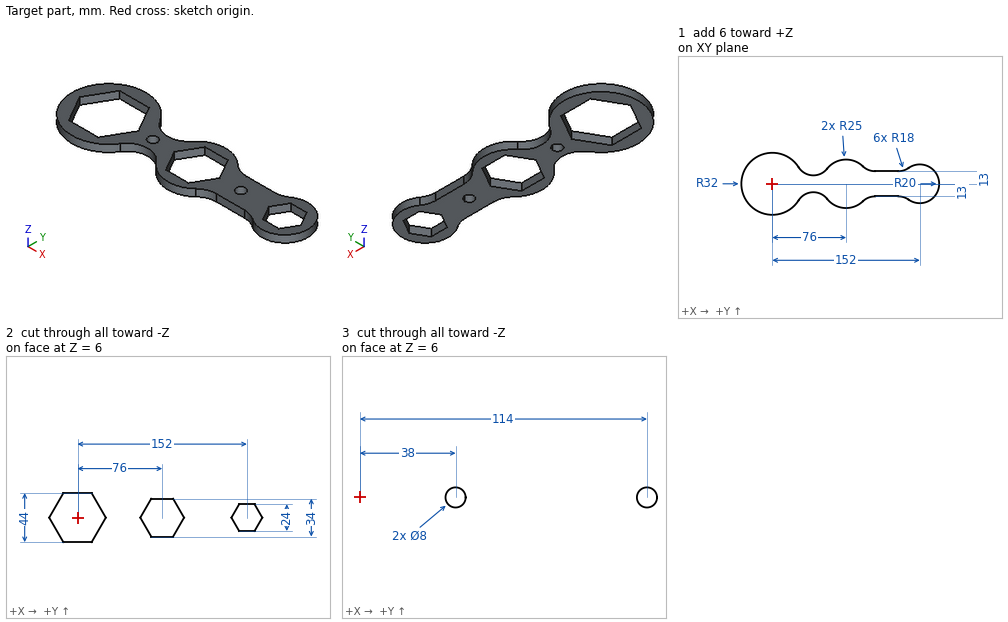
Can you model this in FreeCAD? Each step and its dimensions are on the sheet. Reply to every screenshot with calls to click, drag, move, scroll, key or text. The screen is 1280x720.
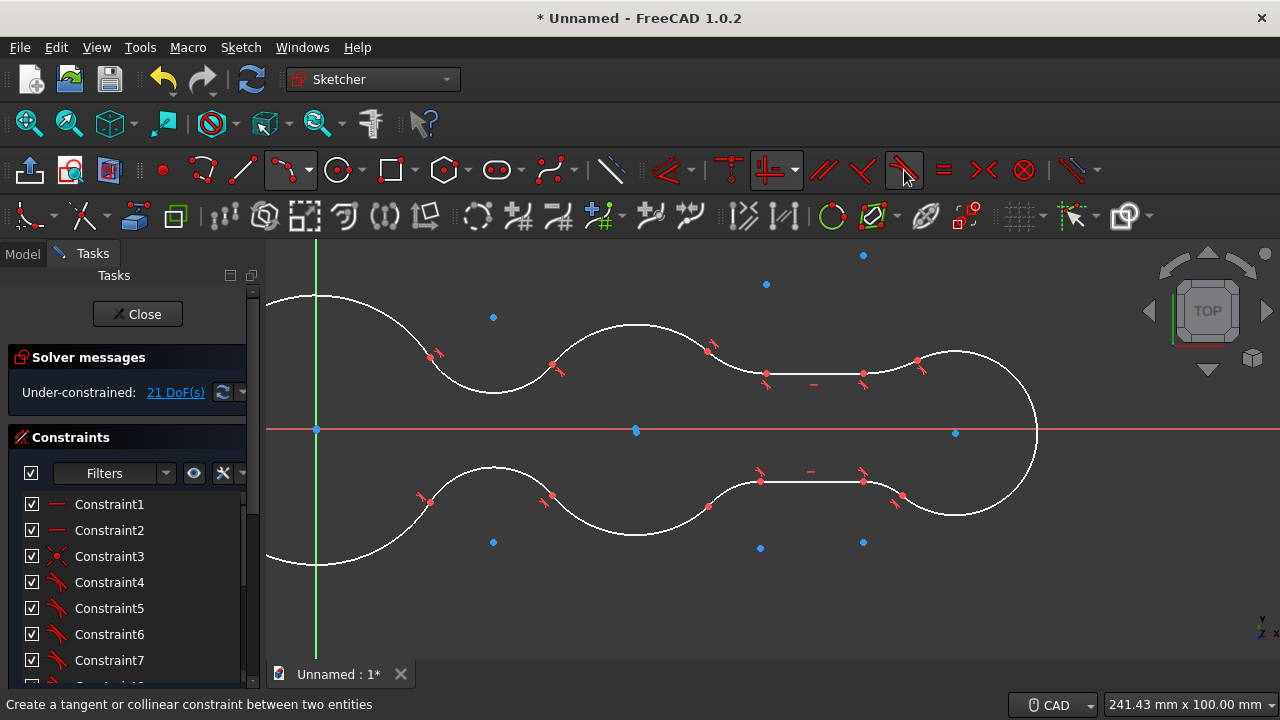
click(594, 527)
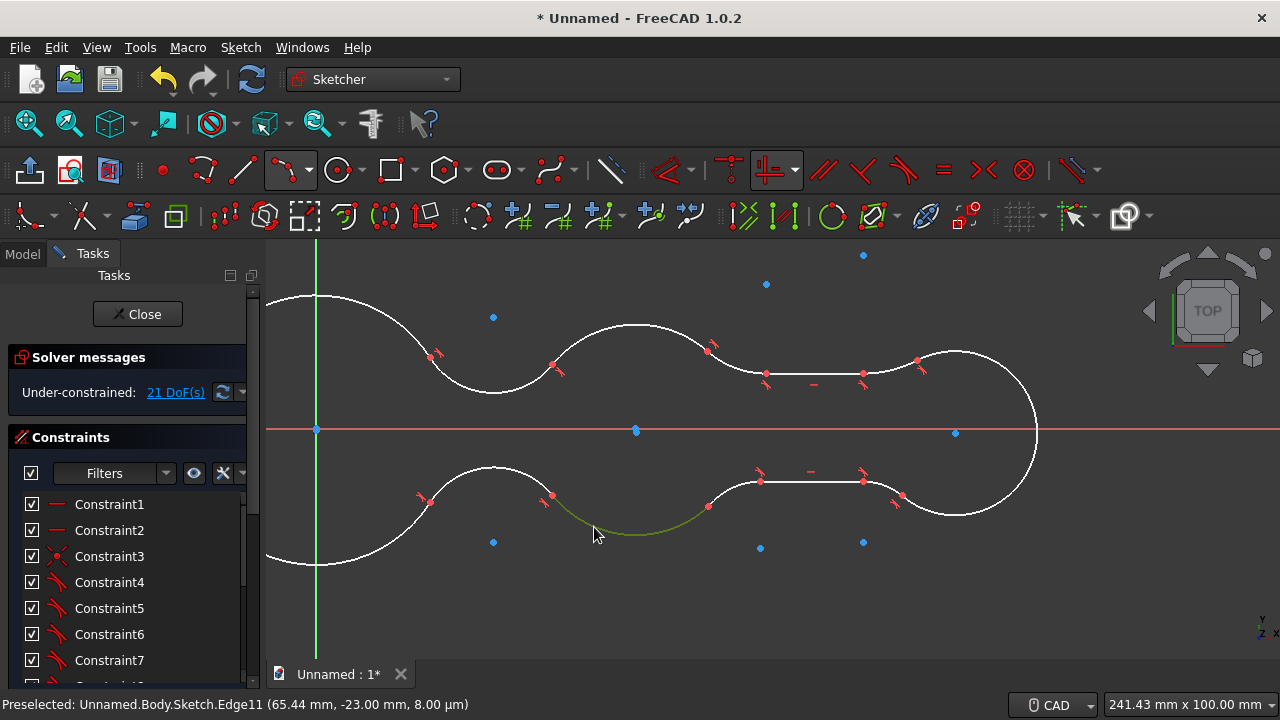
click(743, 484)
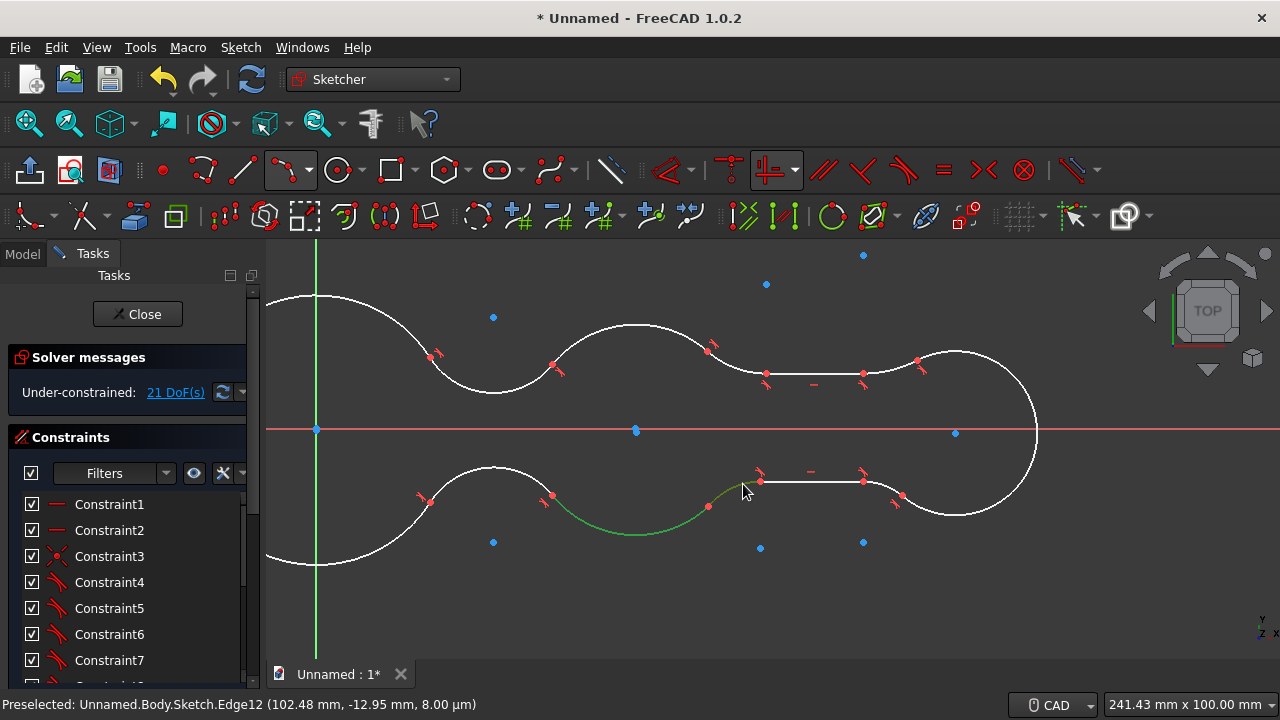
click(904, 170)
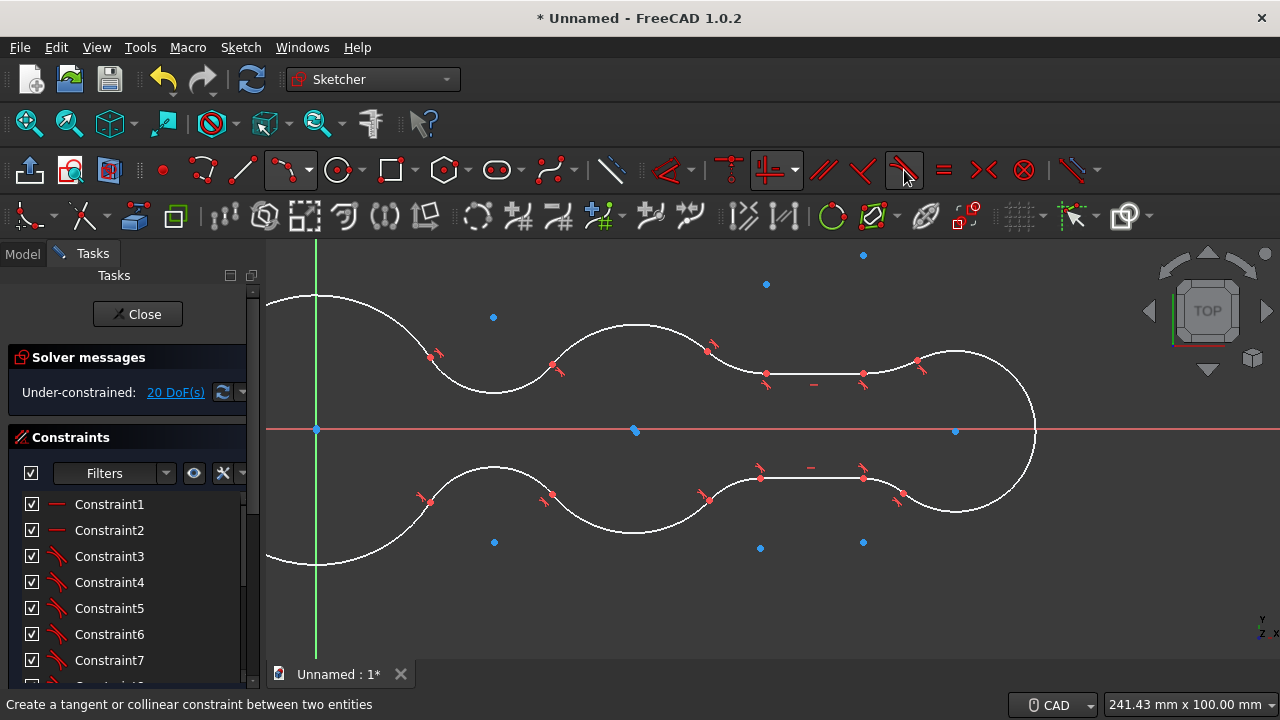
click(662, 328)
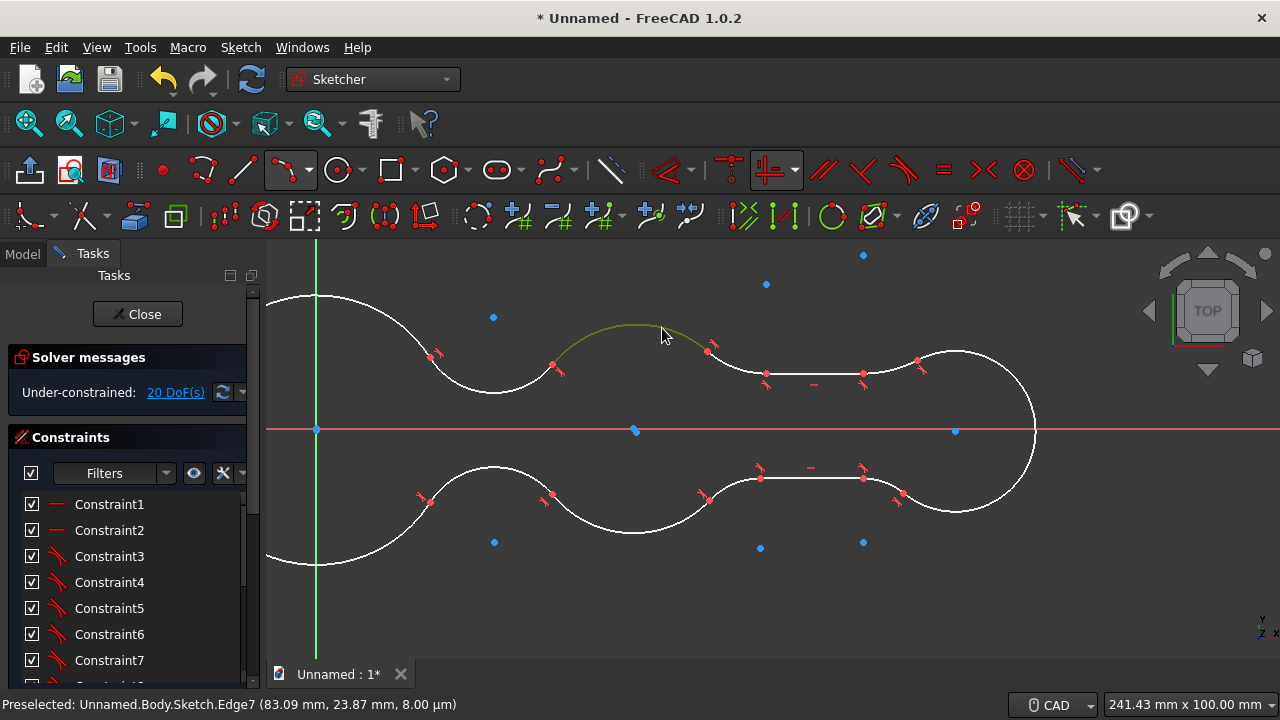
click(595, 526)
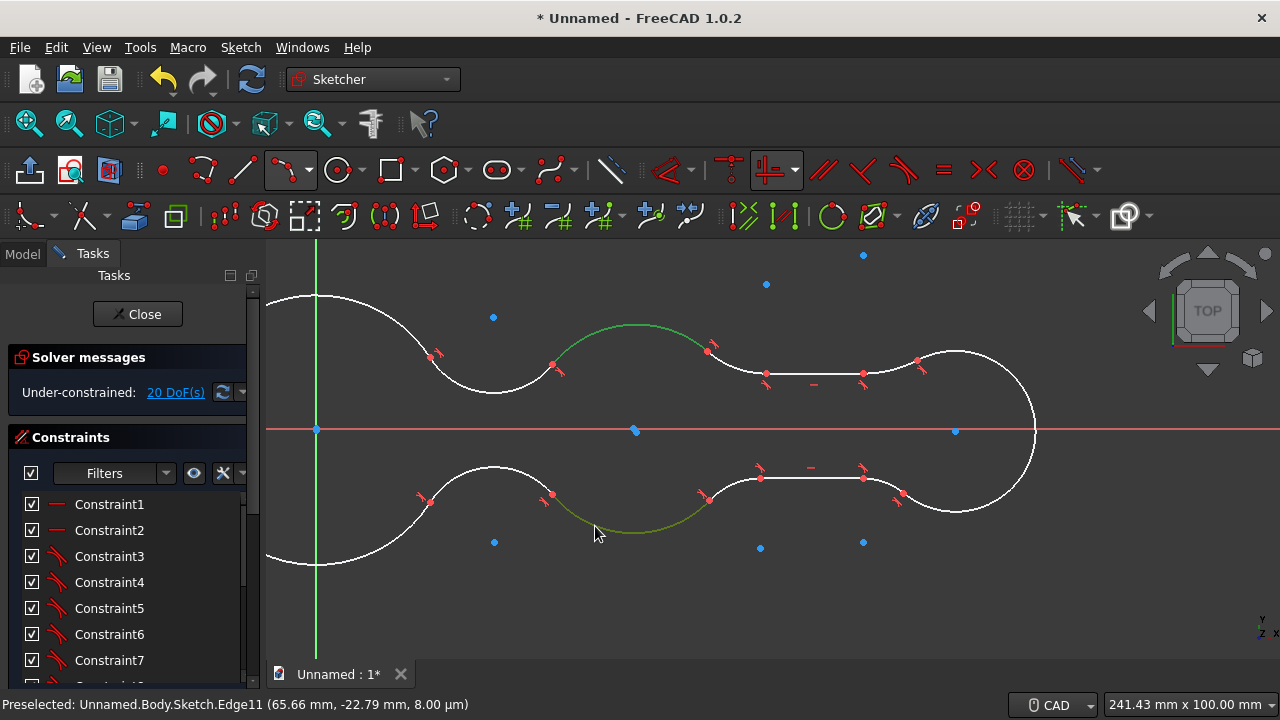
click(730, 170)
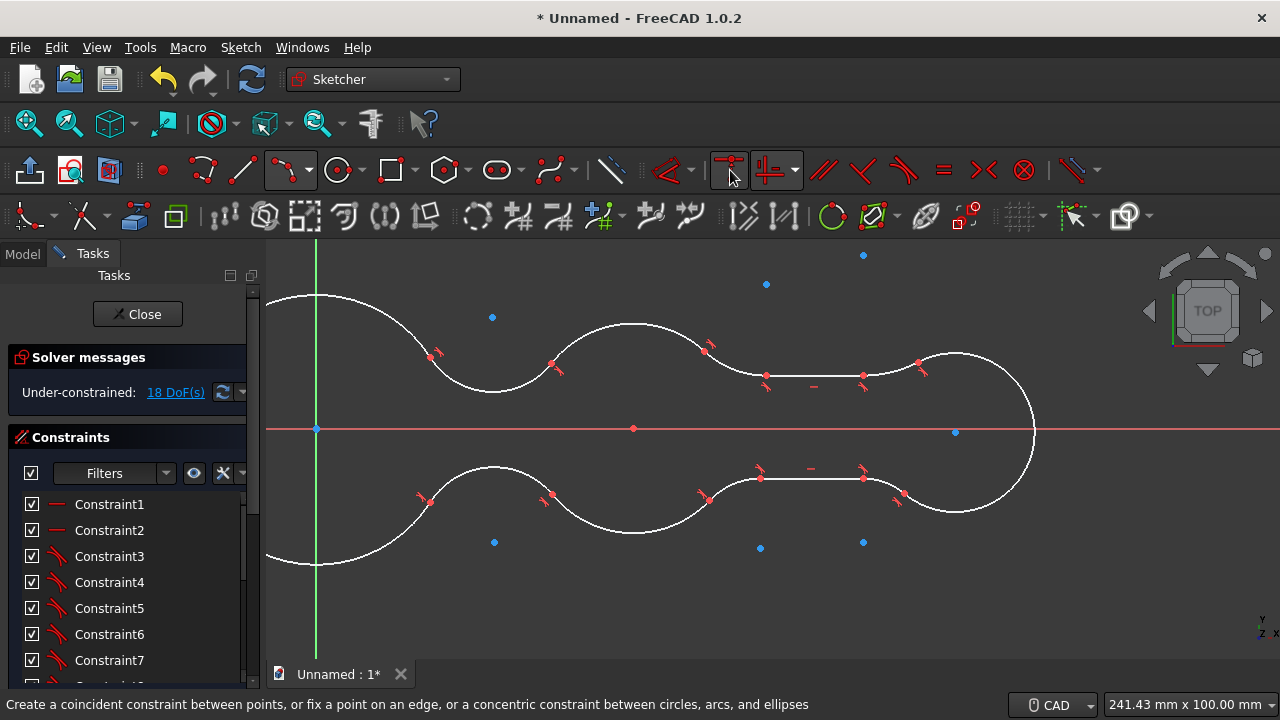
drag(306, 419, 326, 440)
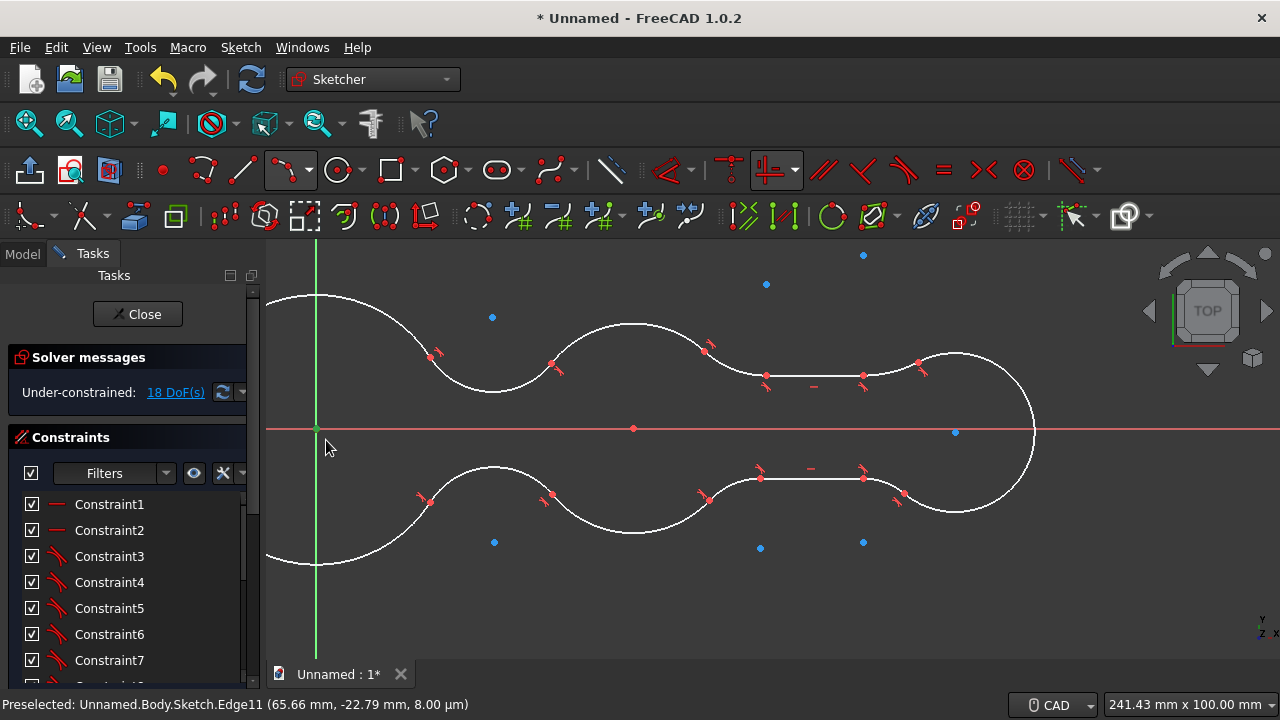
click(730, 170)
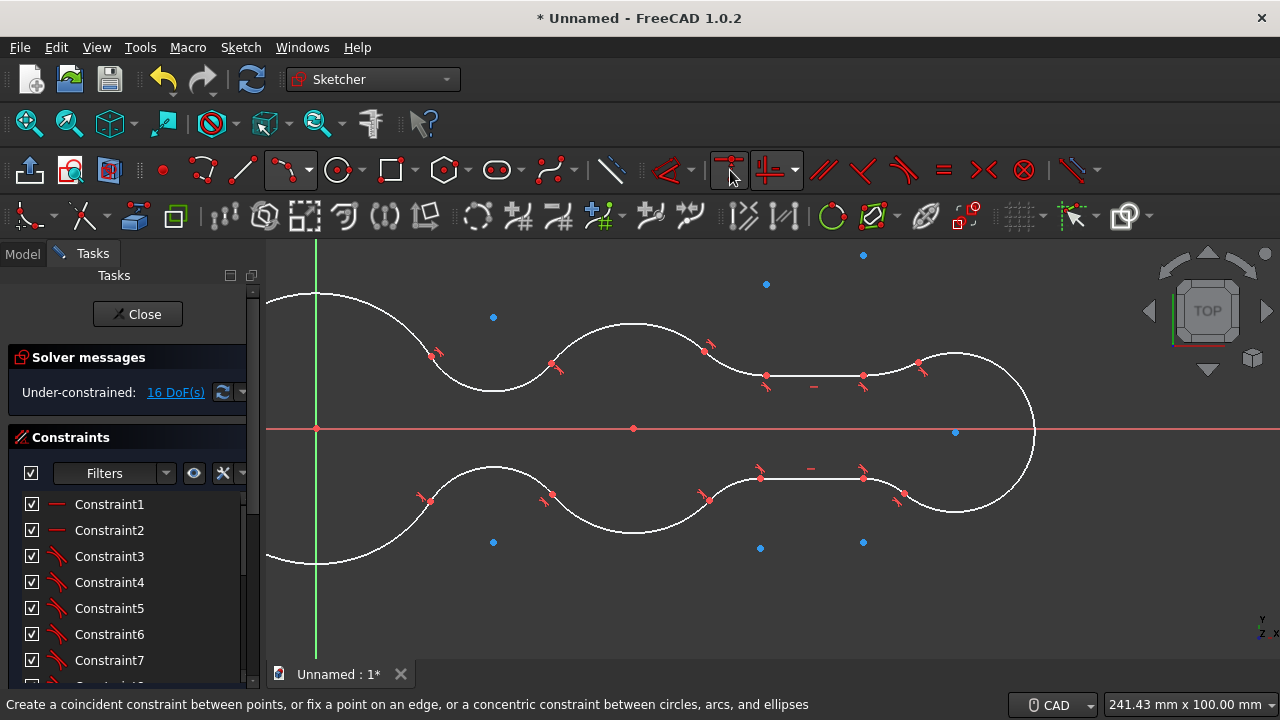
click(893, 486)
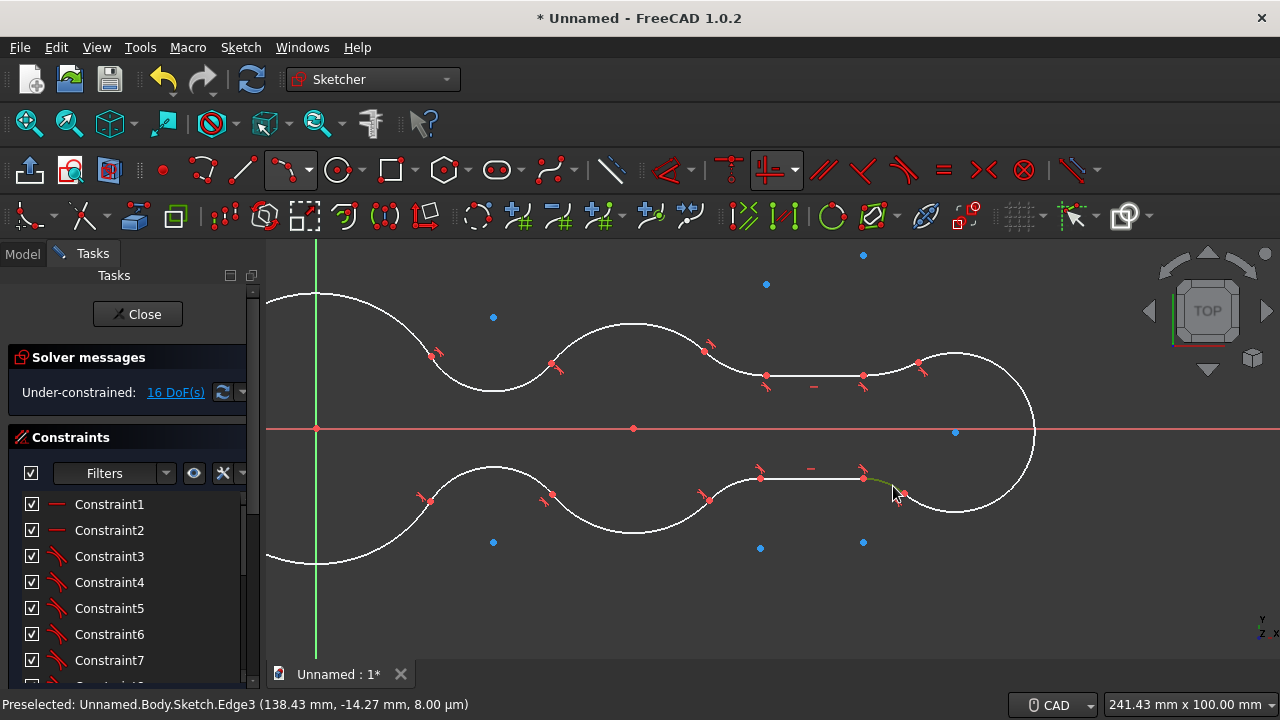
click(880, 374)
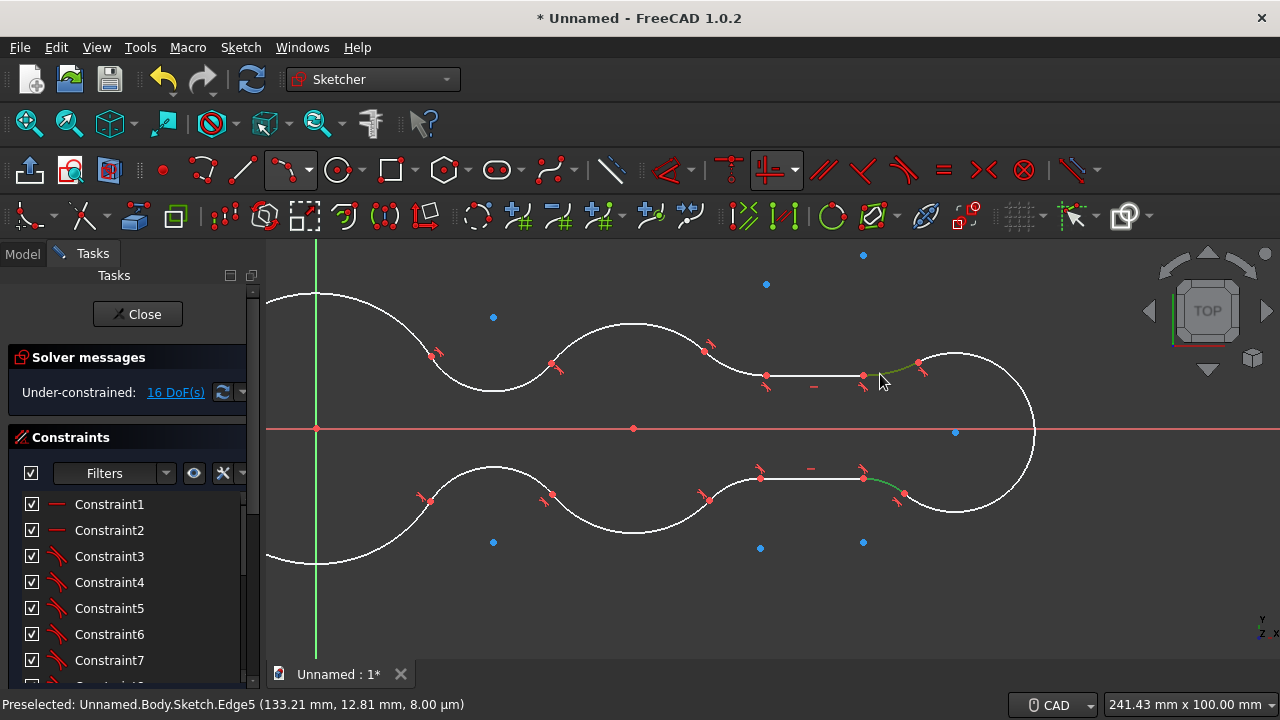
click(721, 363)